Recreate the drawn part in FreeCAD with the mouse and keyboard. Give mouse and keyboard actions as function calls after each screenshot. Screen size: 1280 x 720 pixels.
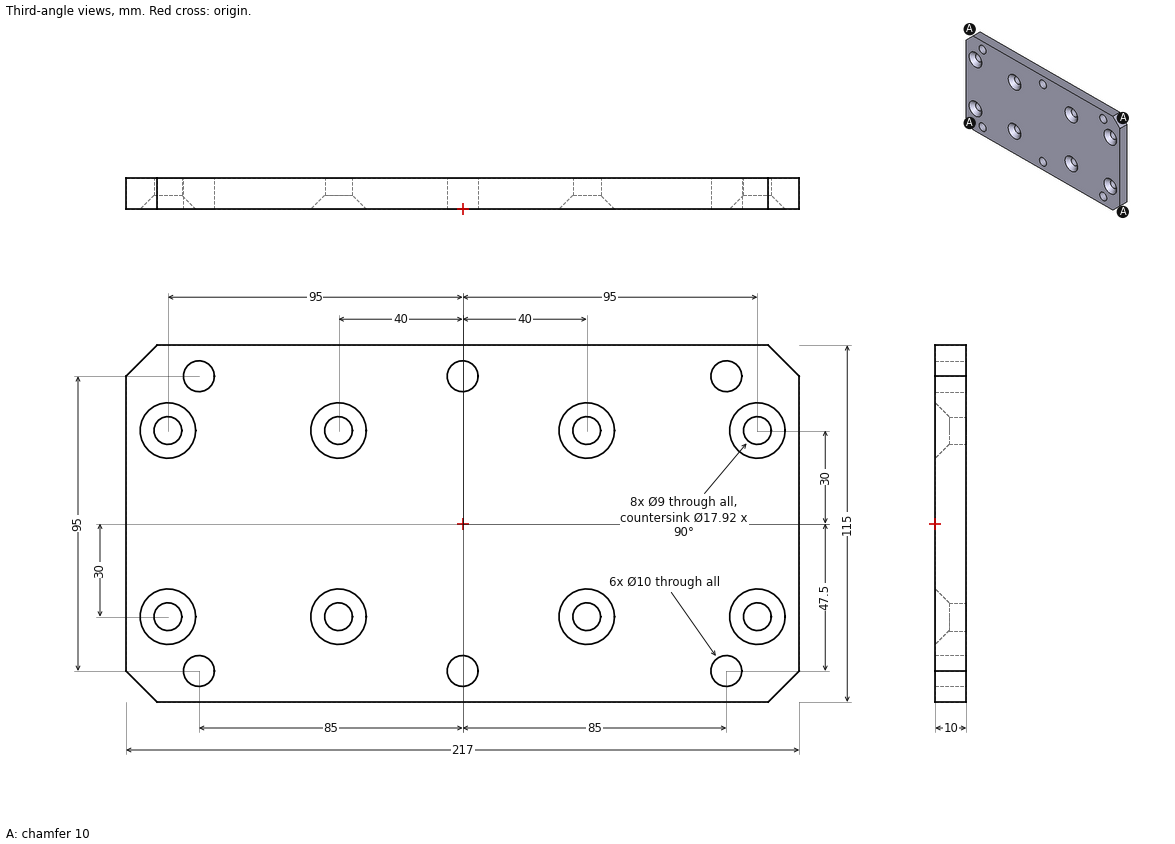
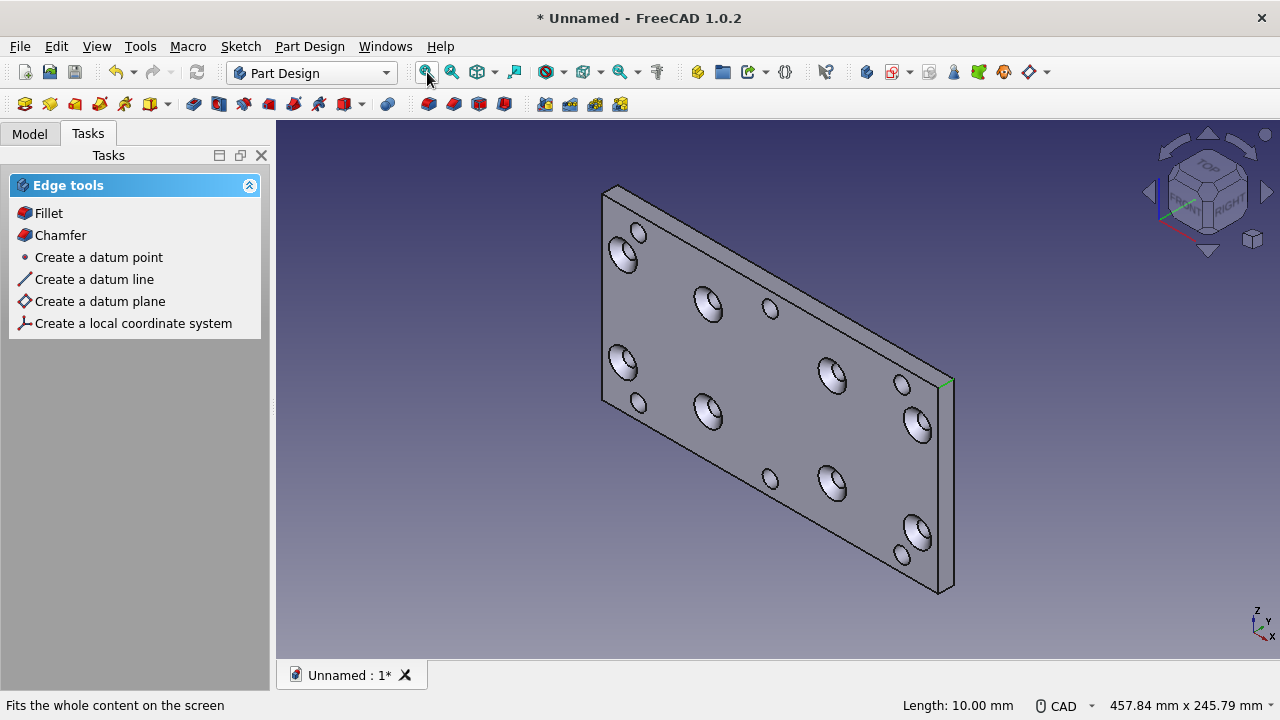
scroll(610, 188, up, 4)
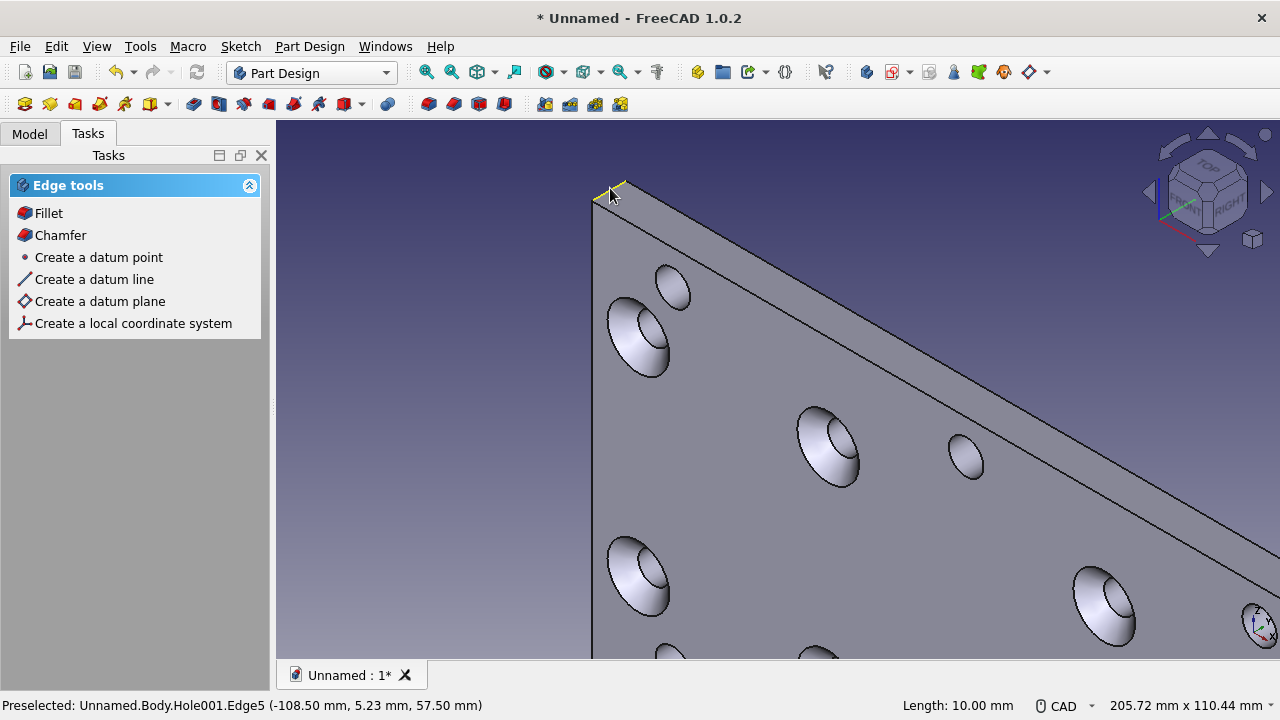
click(427, 72)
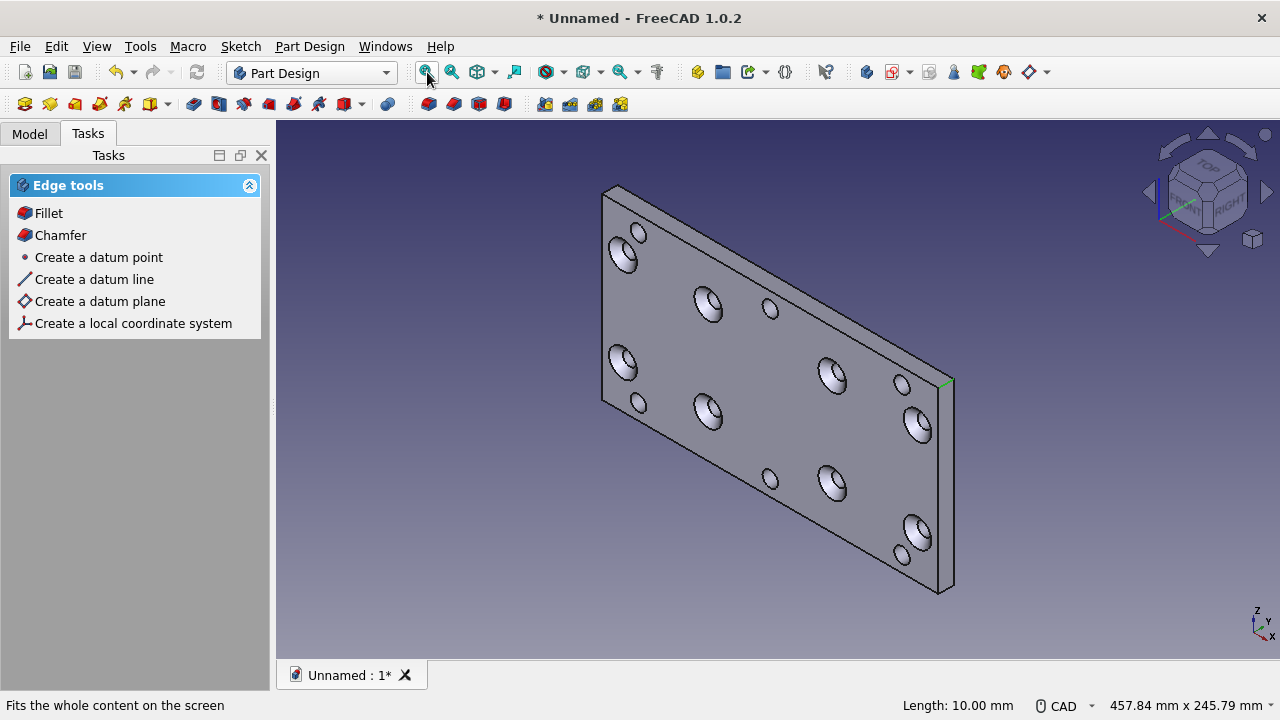
key(2)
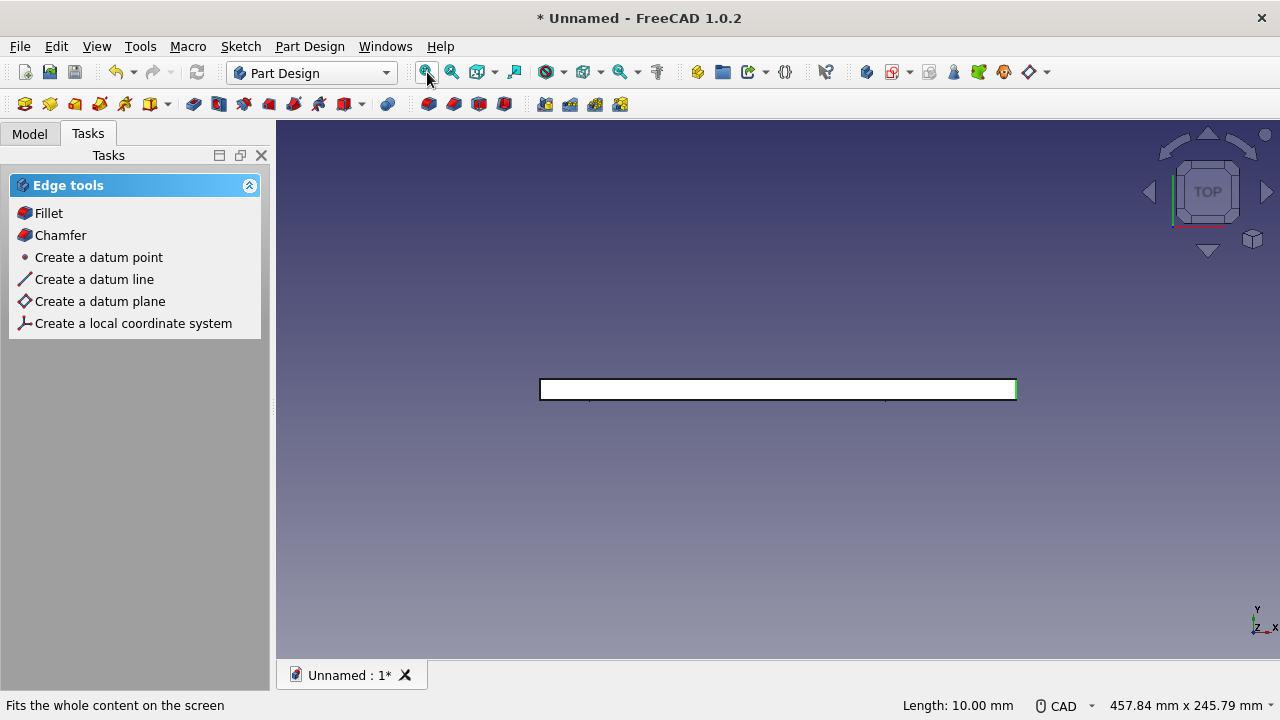
click(540, 388, ctrl)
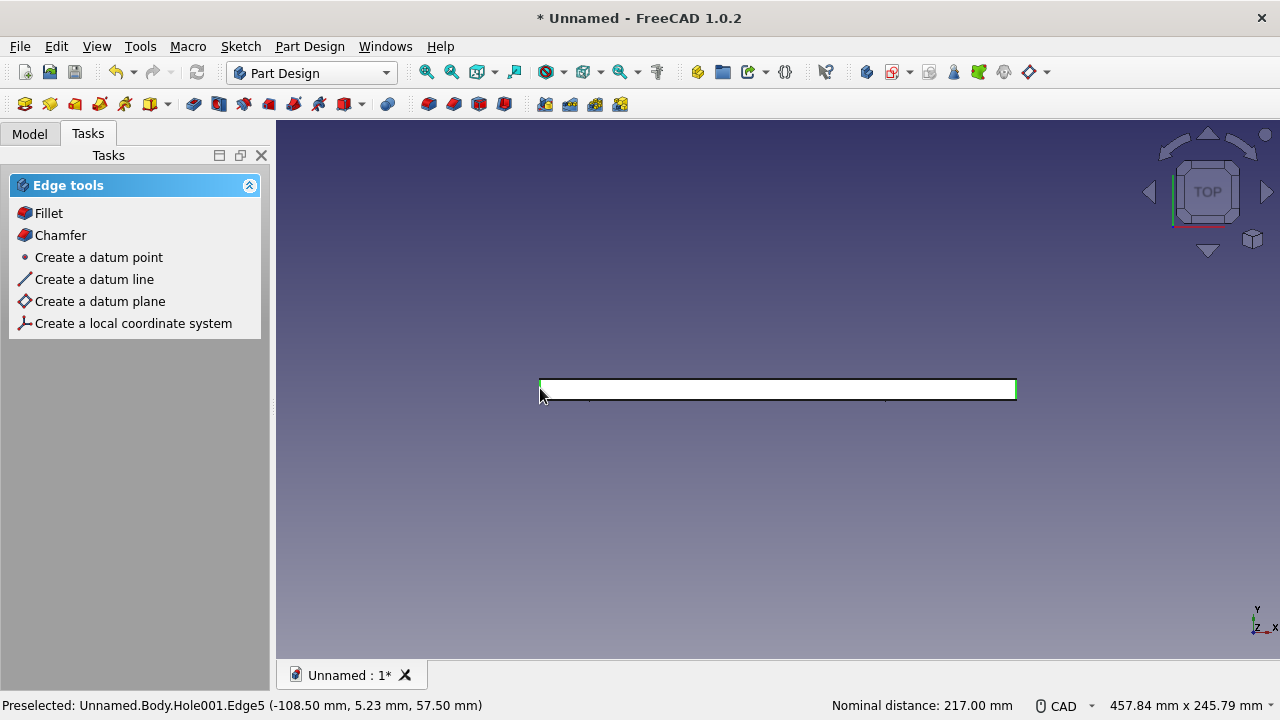
scroll(540, 388, up, 4)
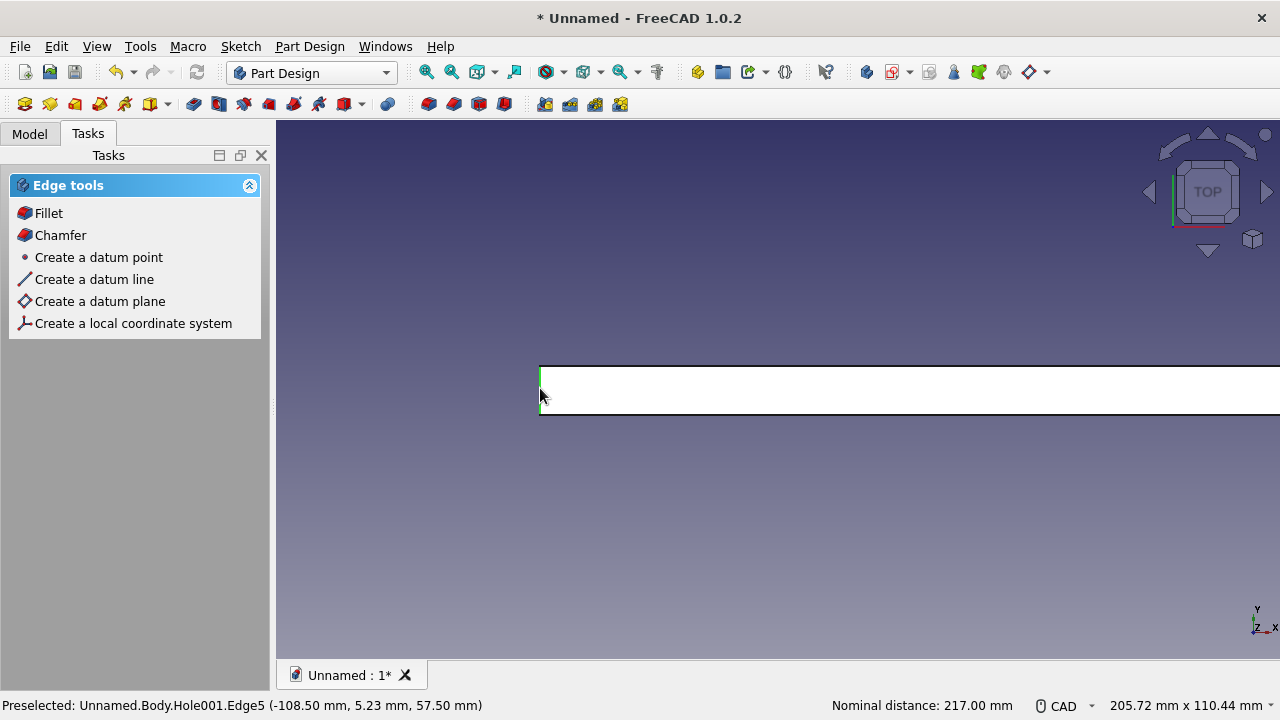
click(427, 72)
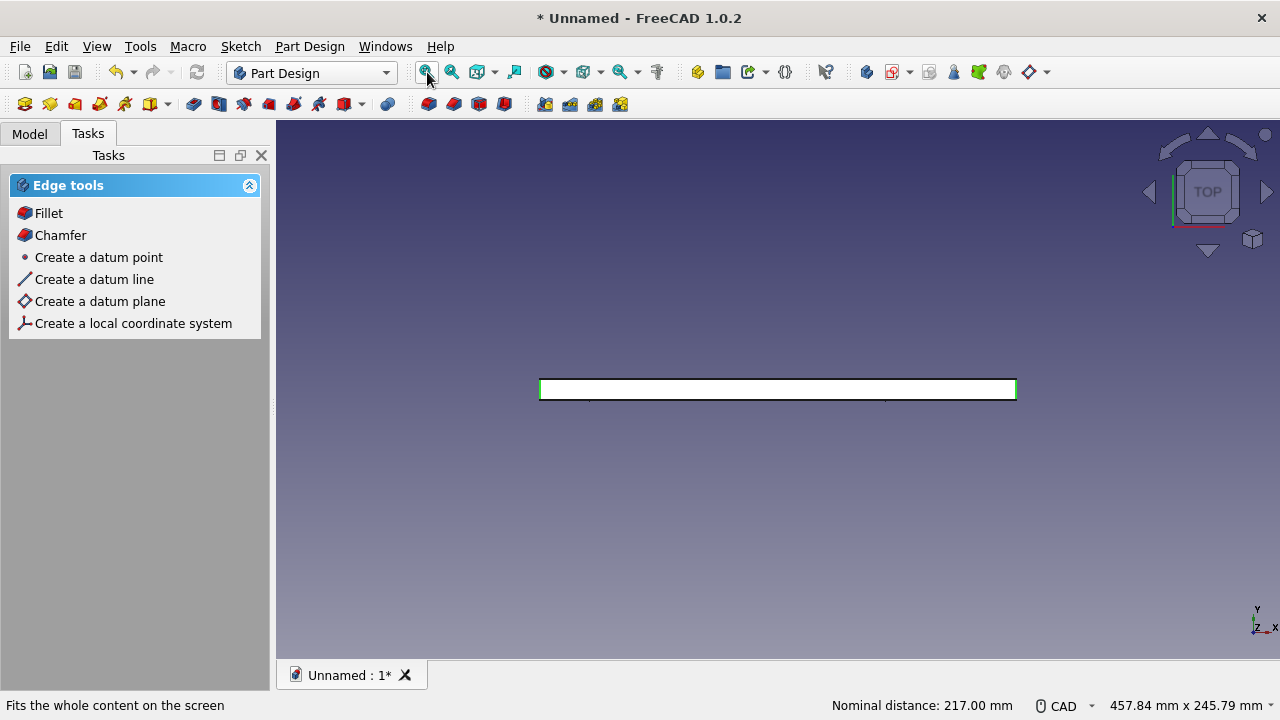
key(1)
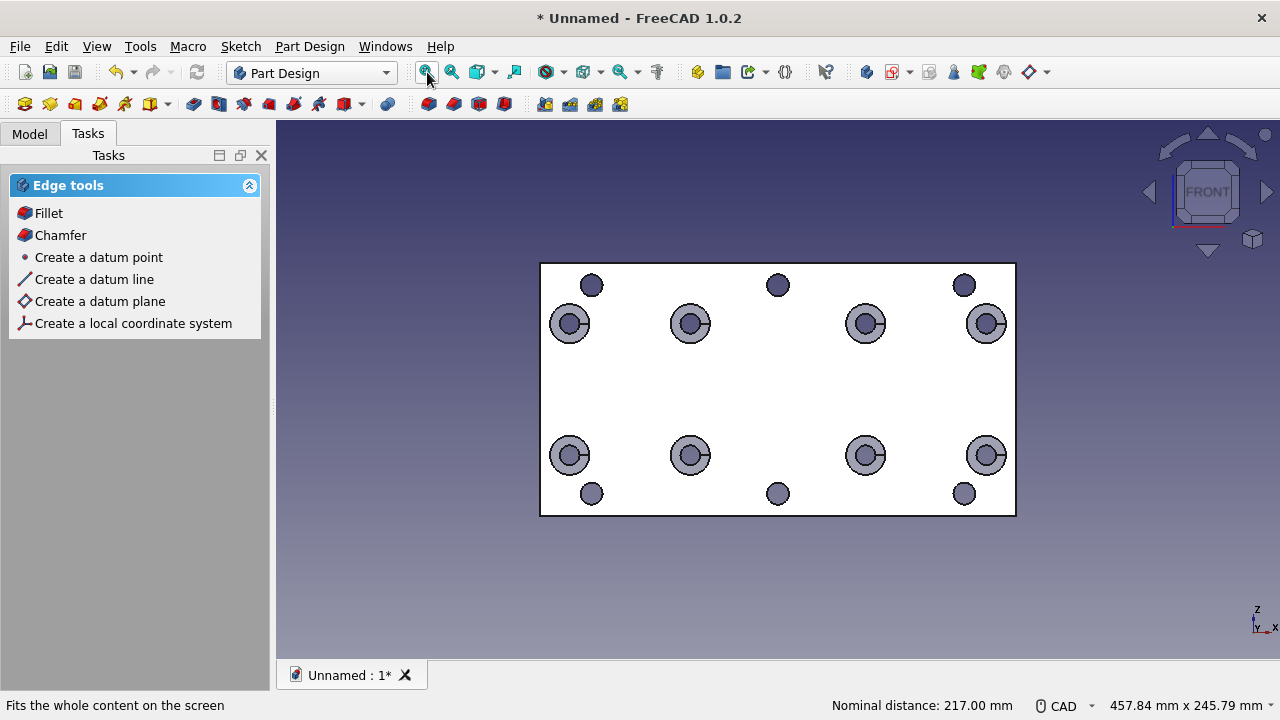
scroll(540, 515, up, 4)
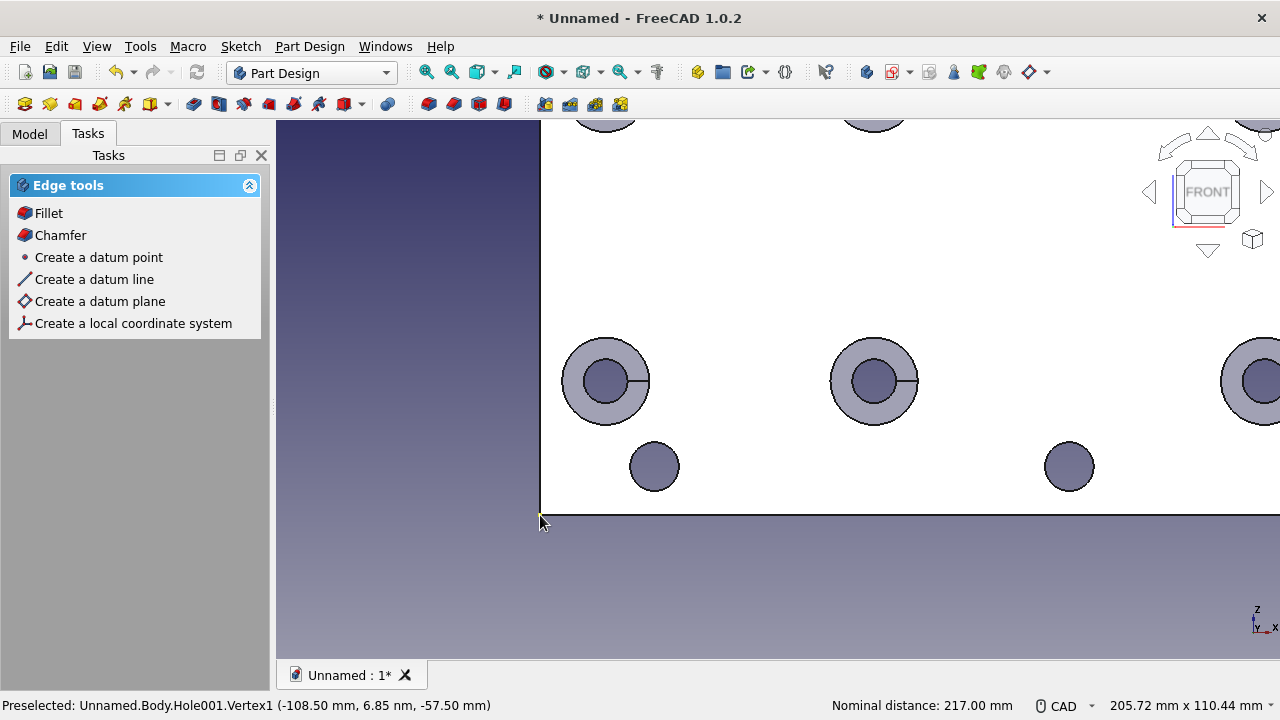
click(427, 72)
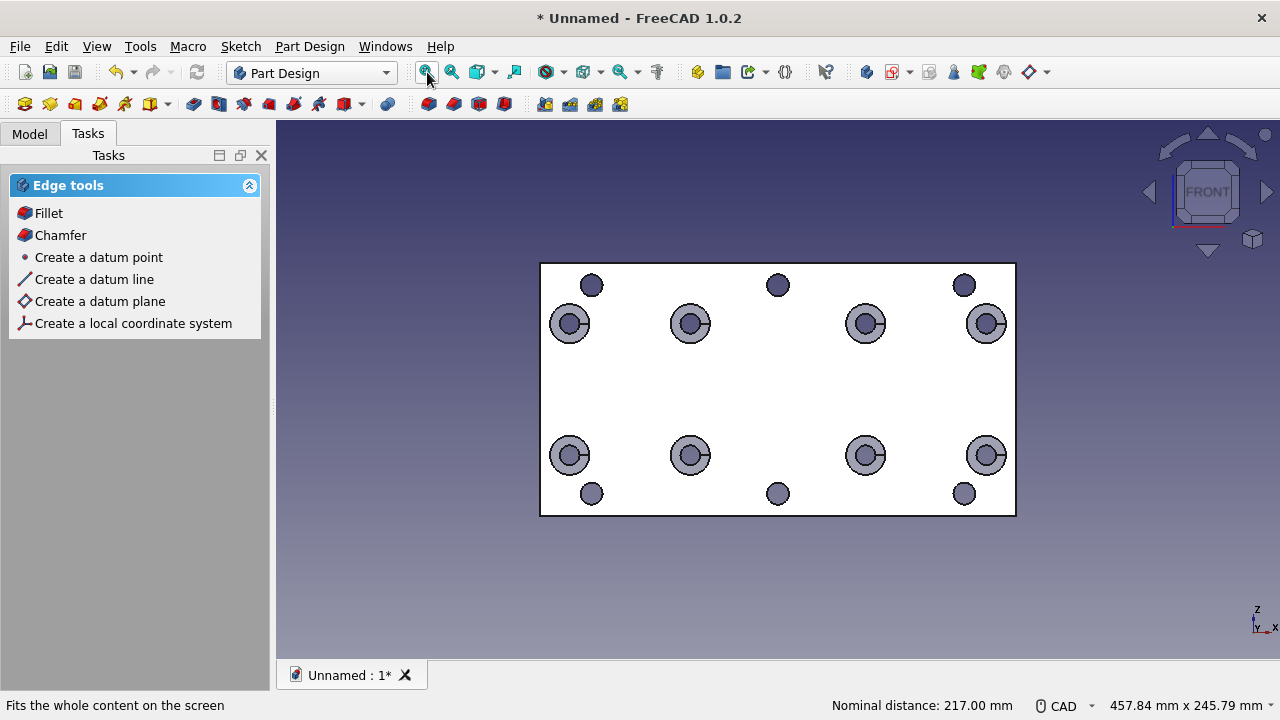
key(3)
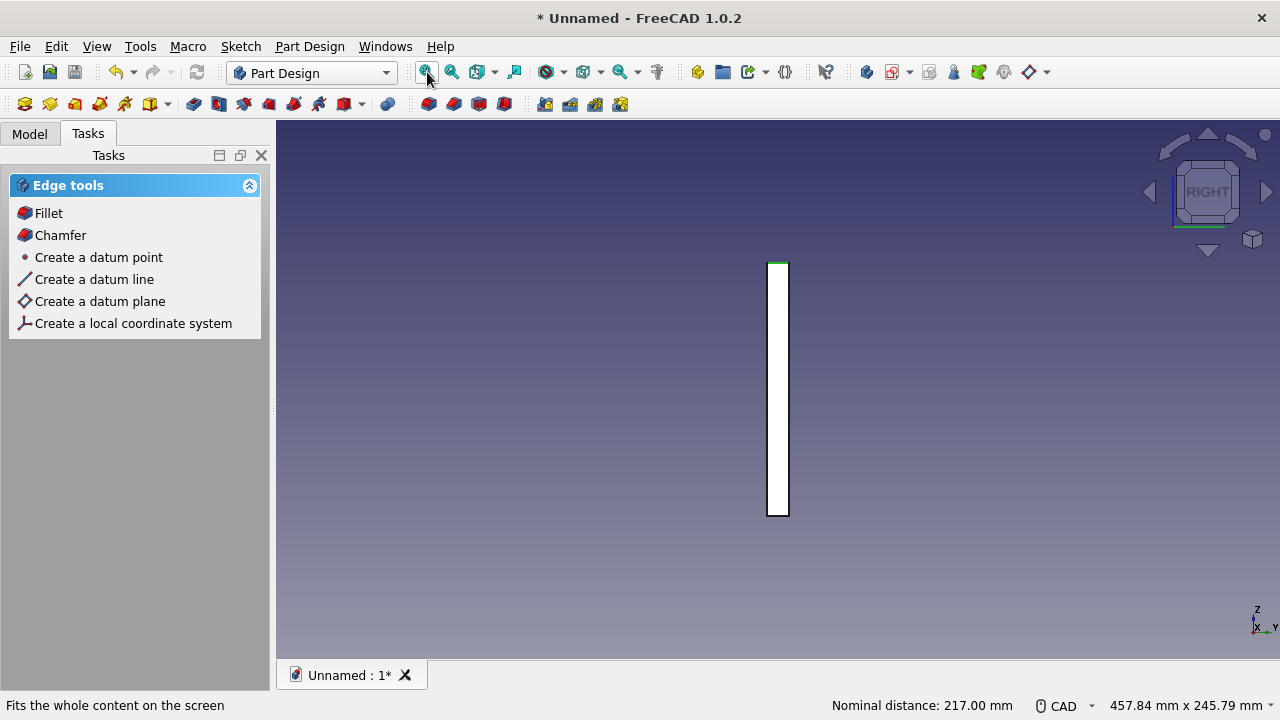
click(778, 515, ctrl)